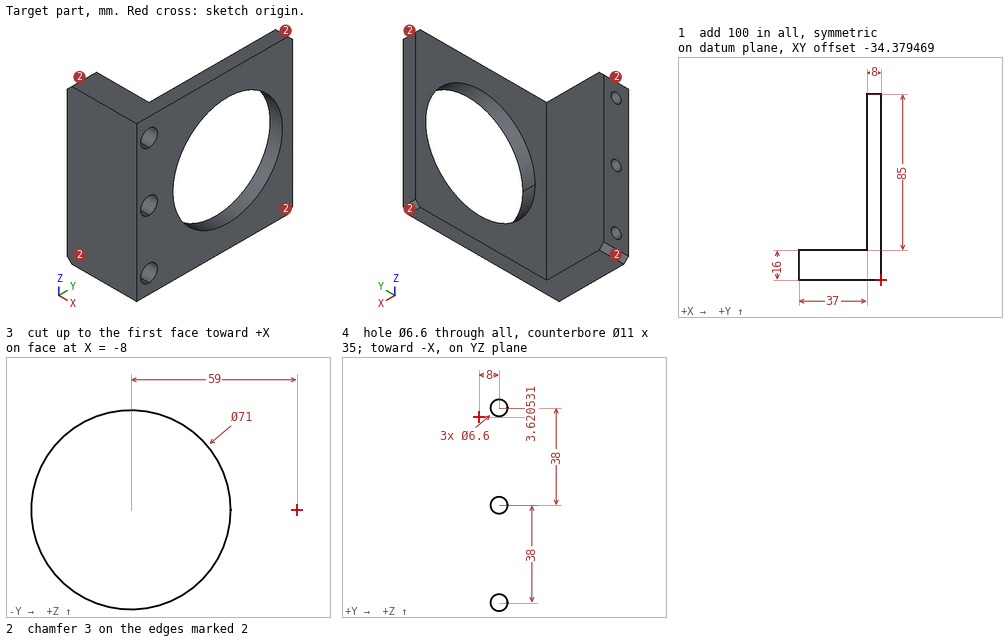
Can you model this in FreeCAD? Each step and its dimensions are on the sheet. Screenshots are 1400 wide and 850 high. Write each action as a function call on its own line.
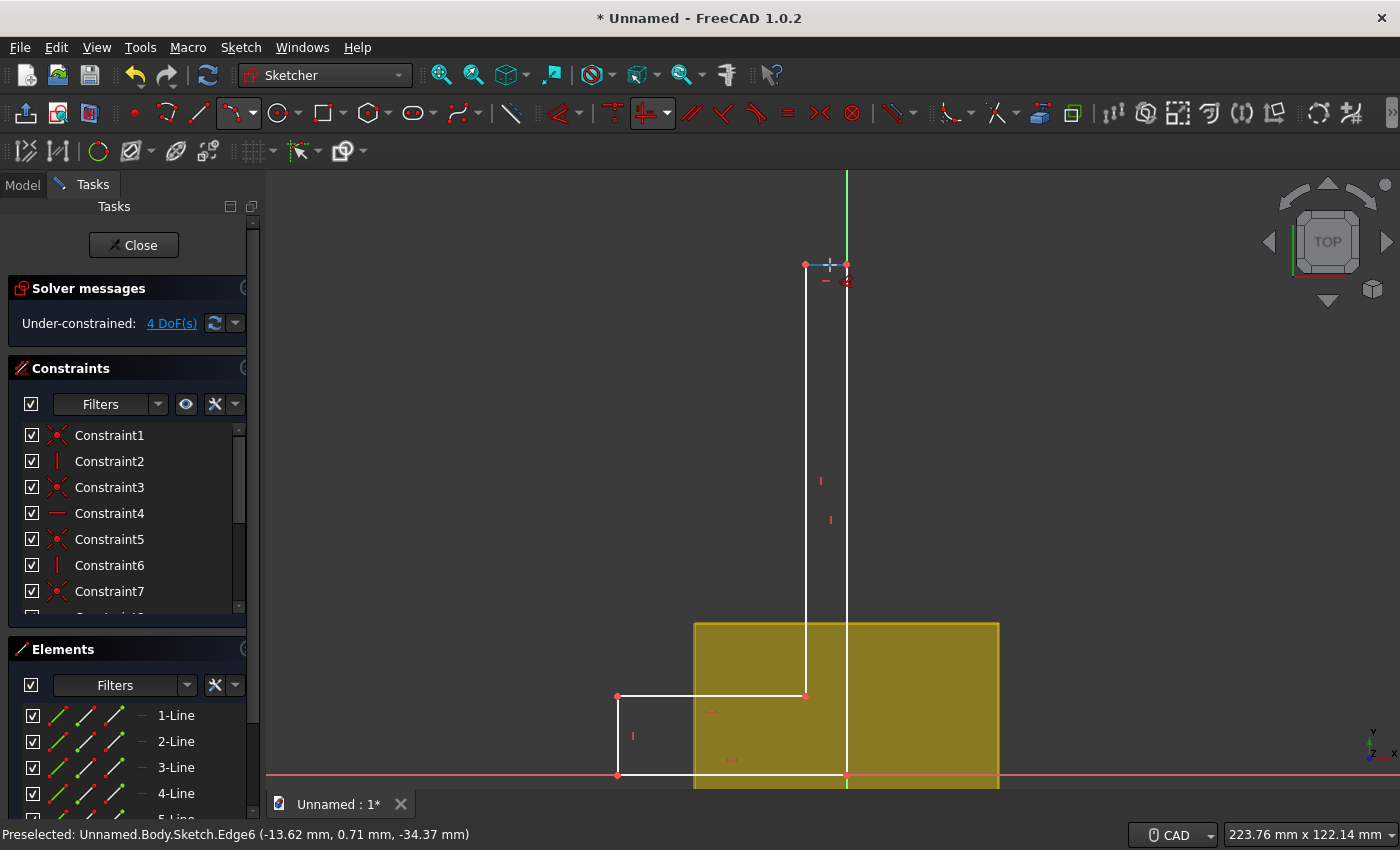
click(830, 265)
click(826, 231)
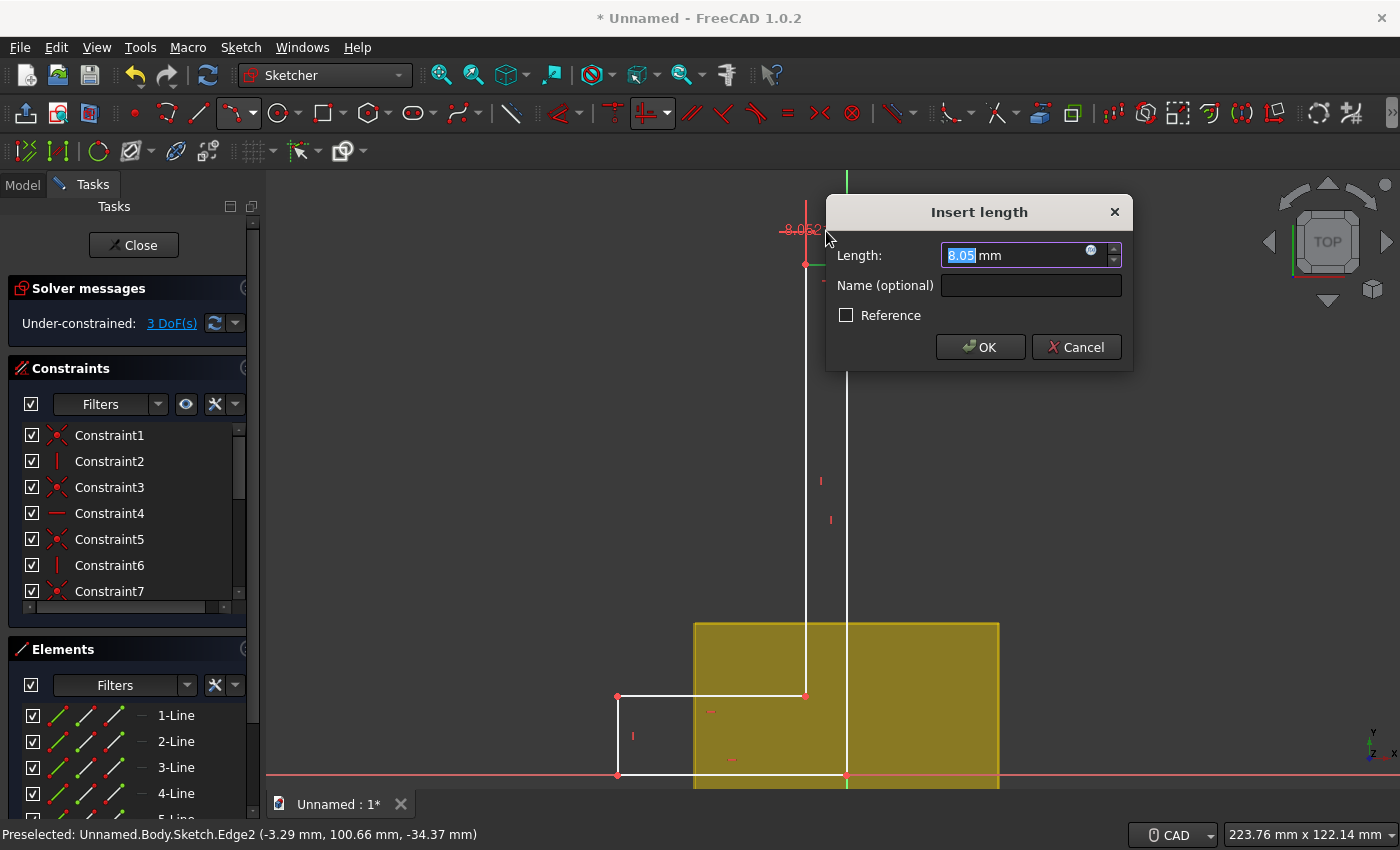
text(8)
key(Return)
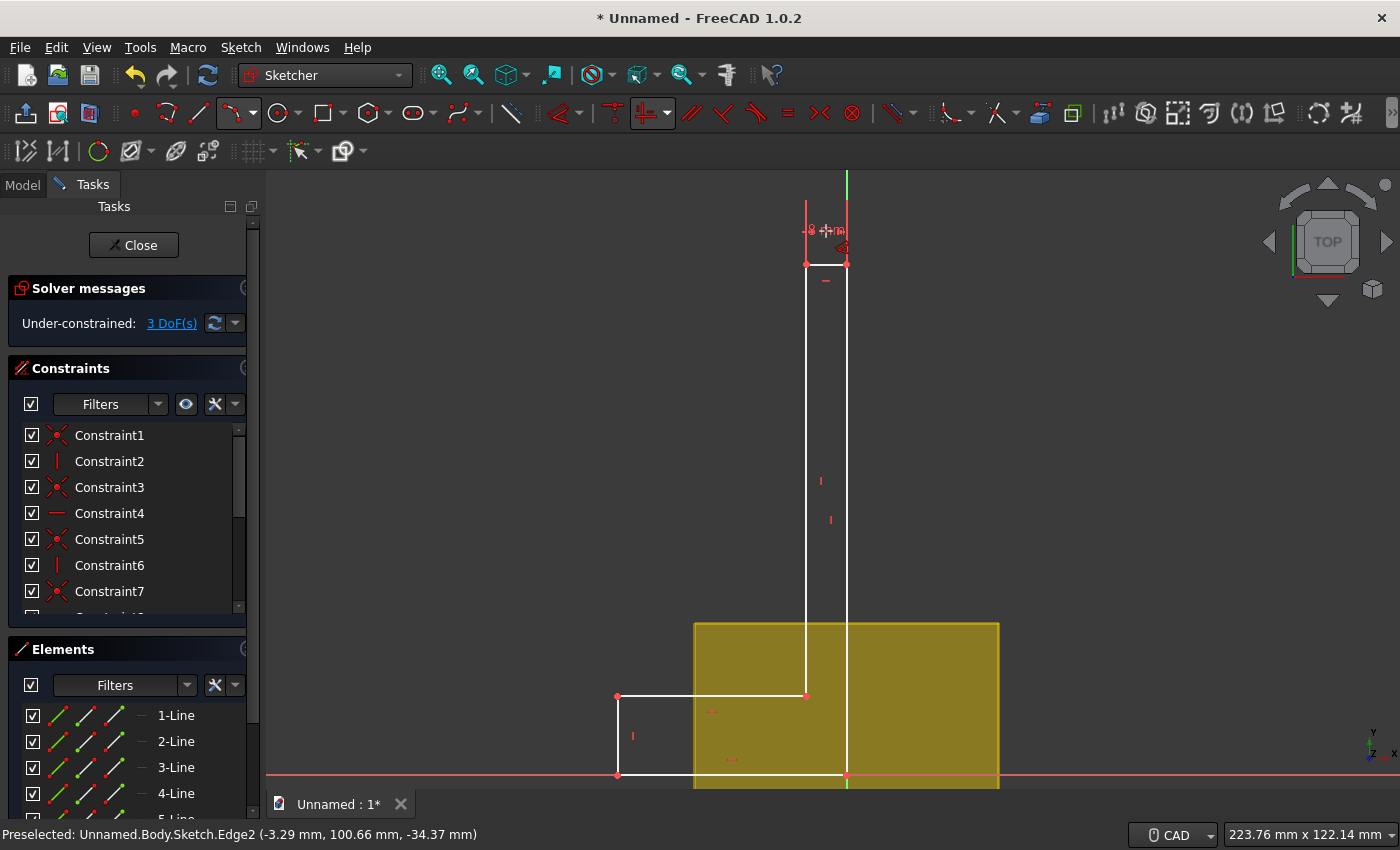
click(806, 394)
click(772, 480)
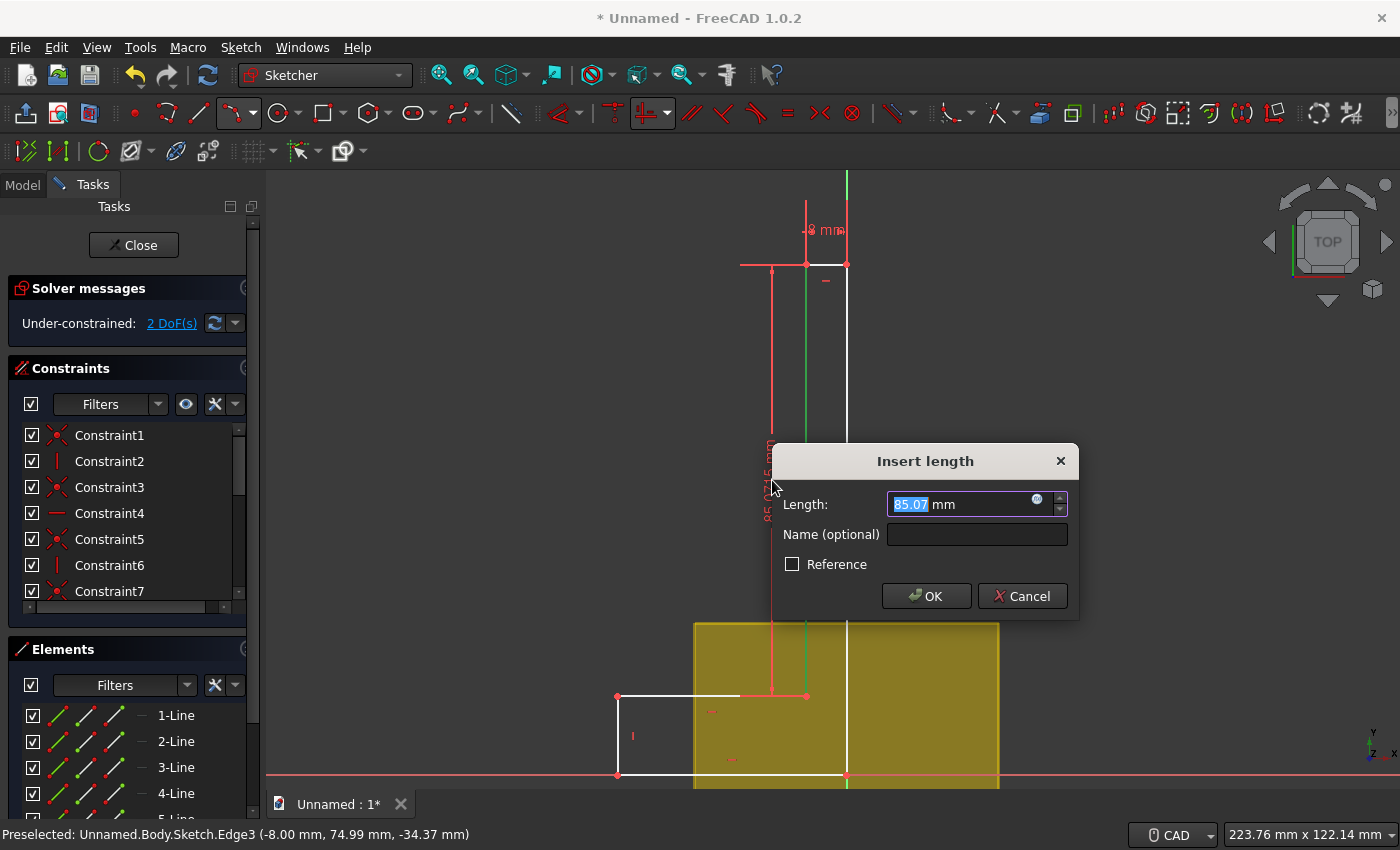
text(85)
key(Return)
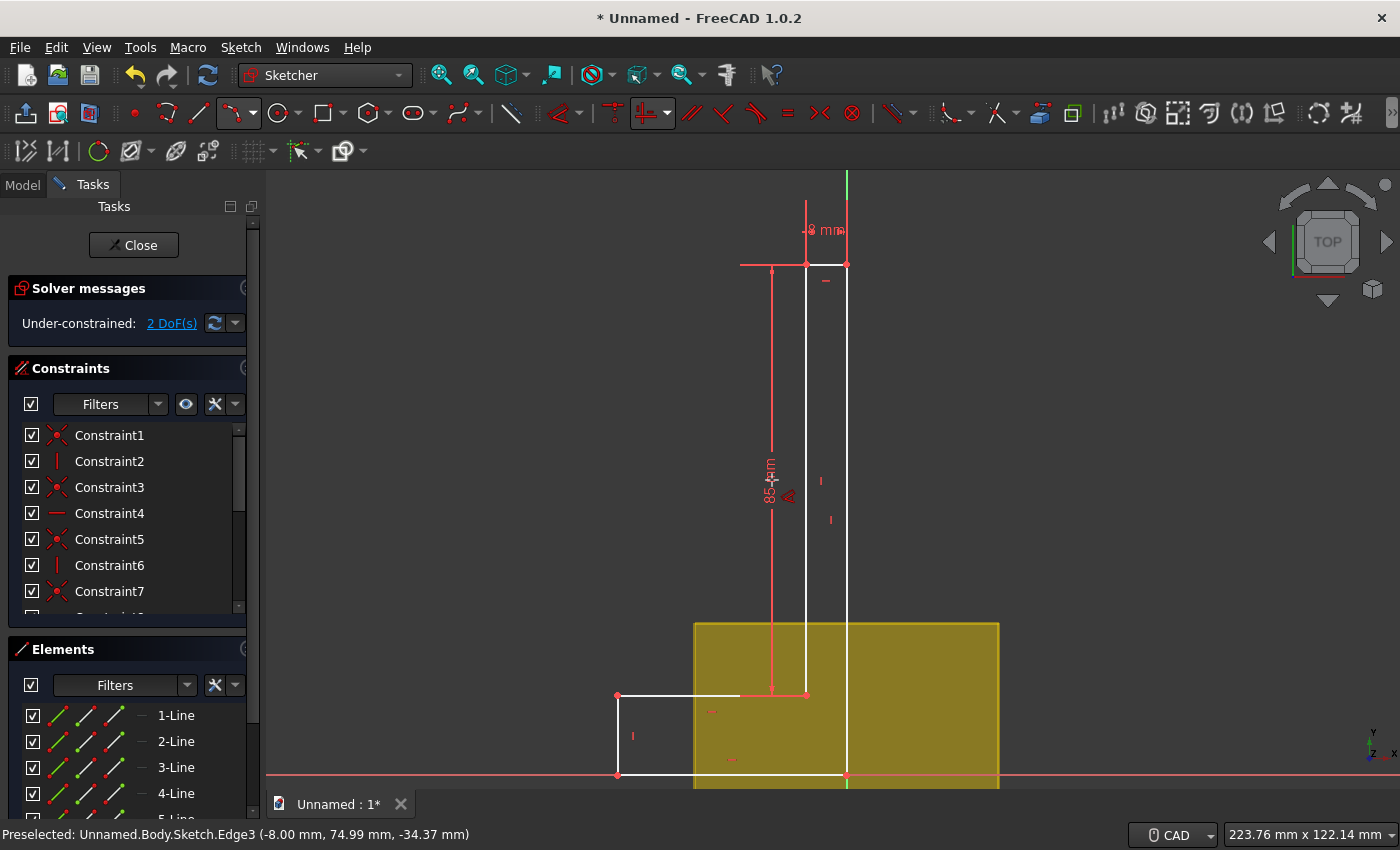
click(750, 696)
click(712, 730)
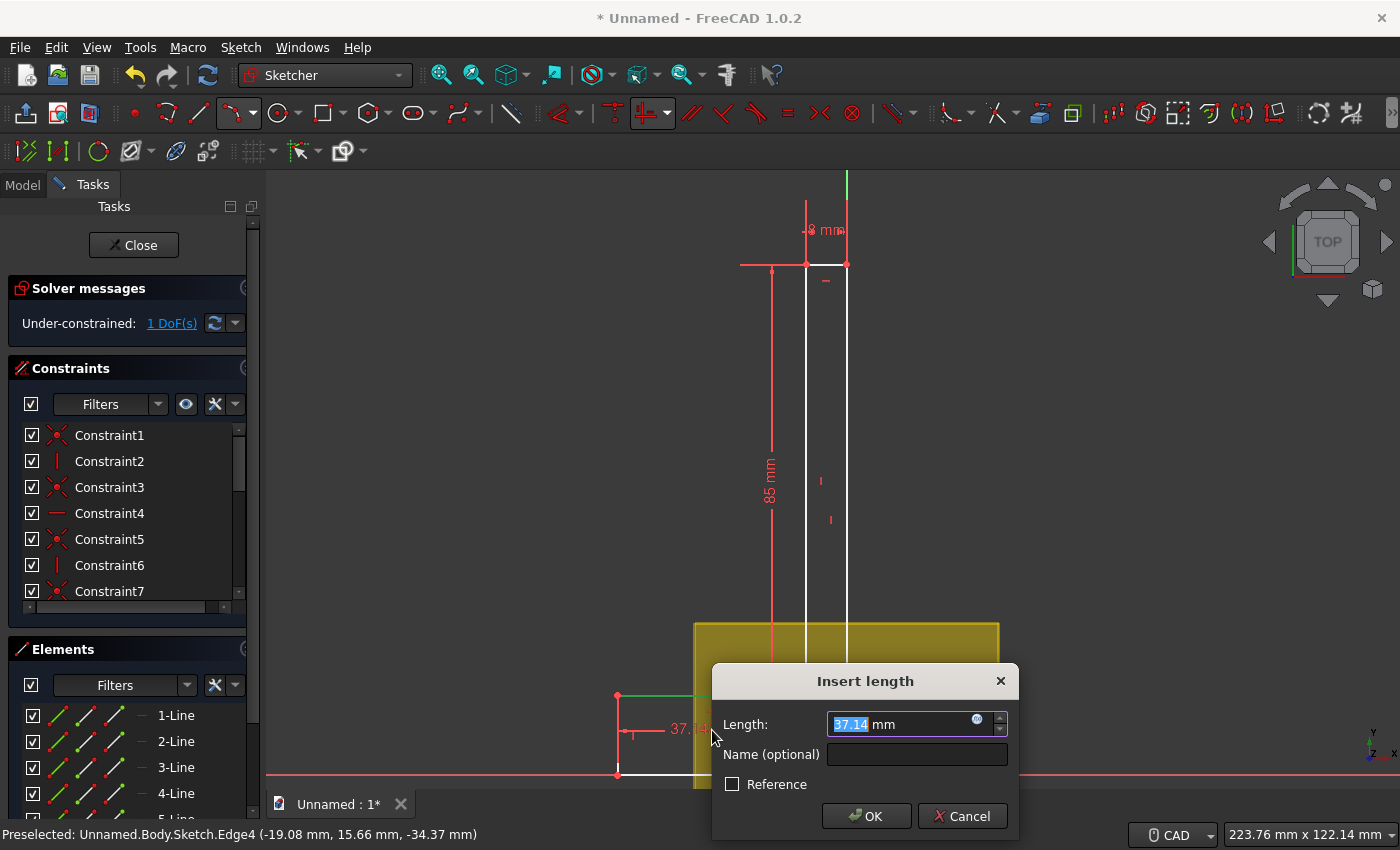
text(37)
key(Return)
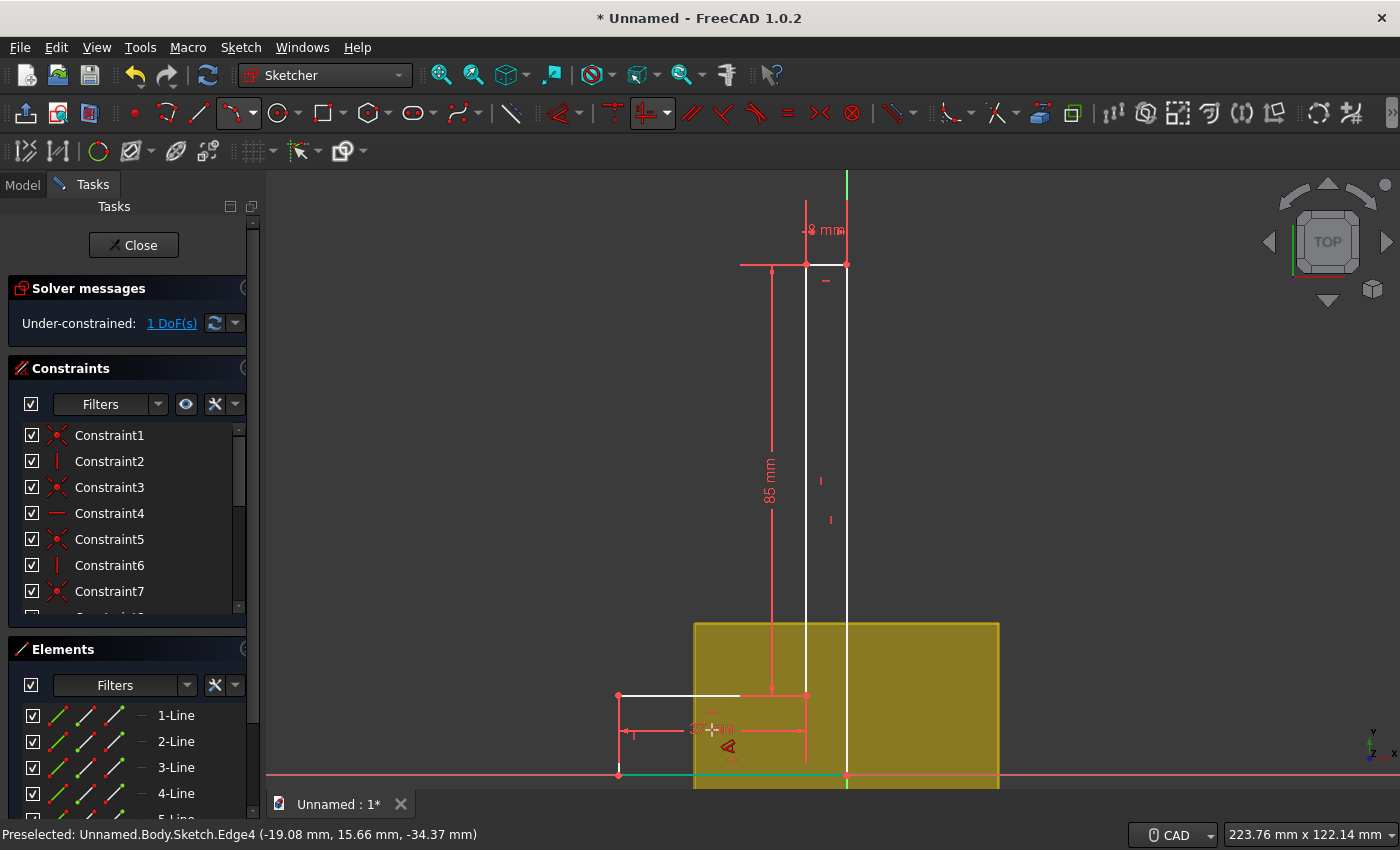
click(619, 720)
click(585, 728)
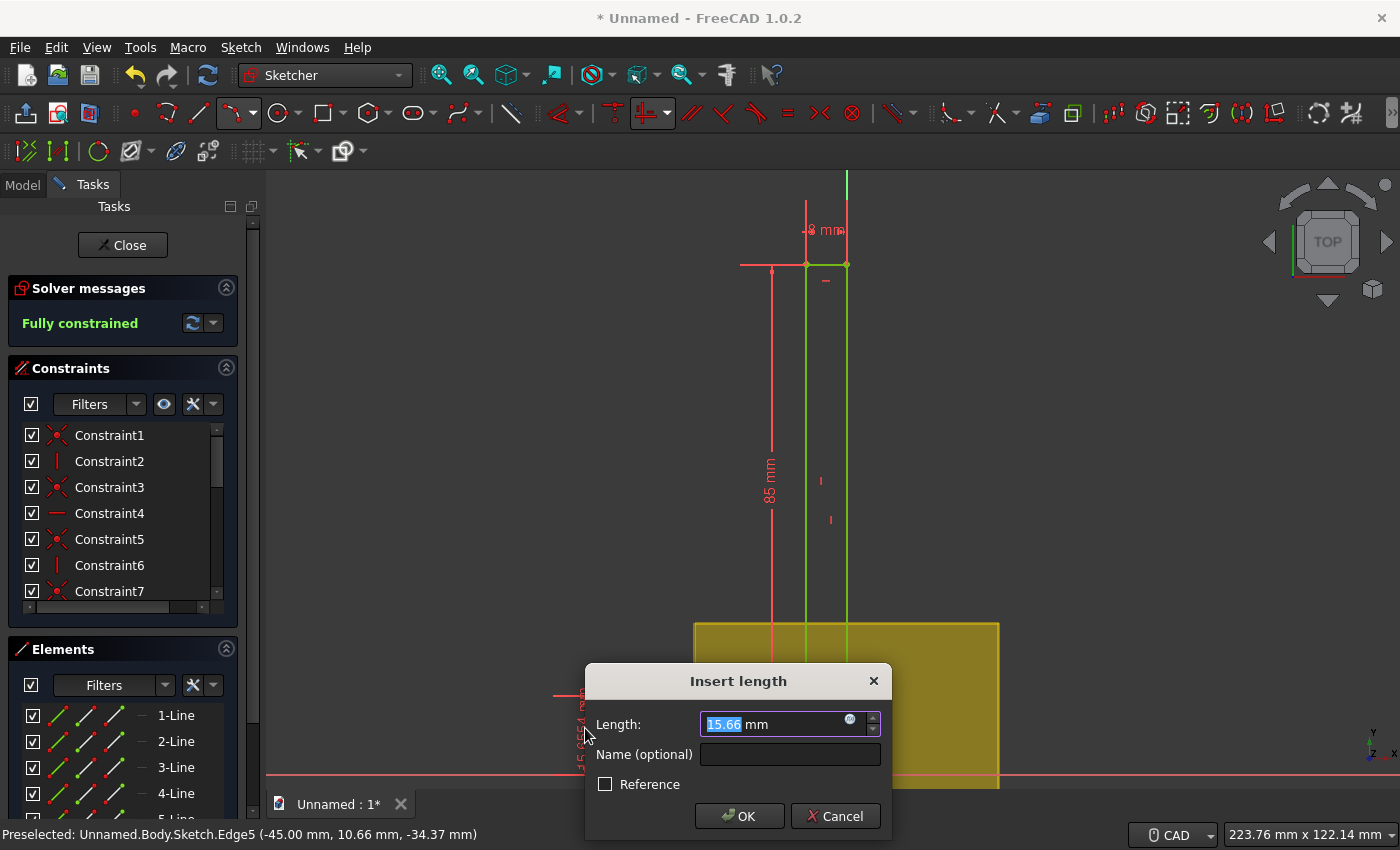
text(16)
key(Return)
key(Escape)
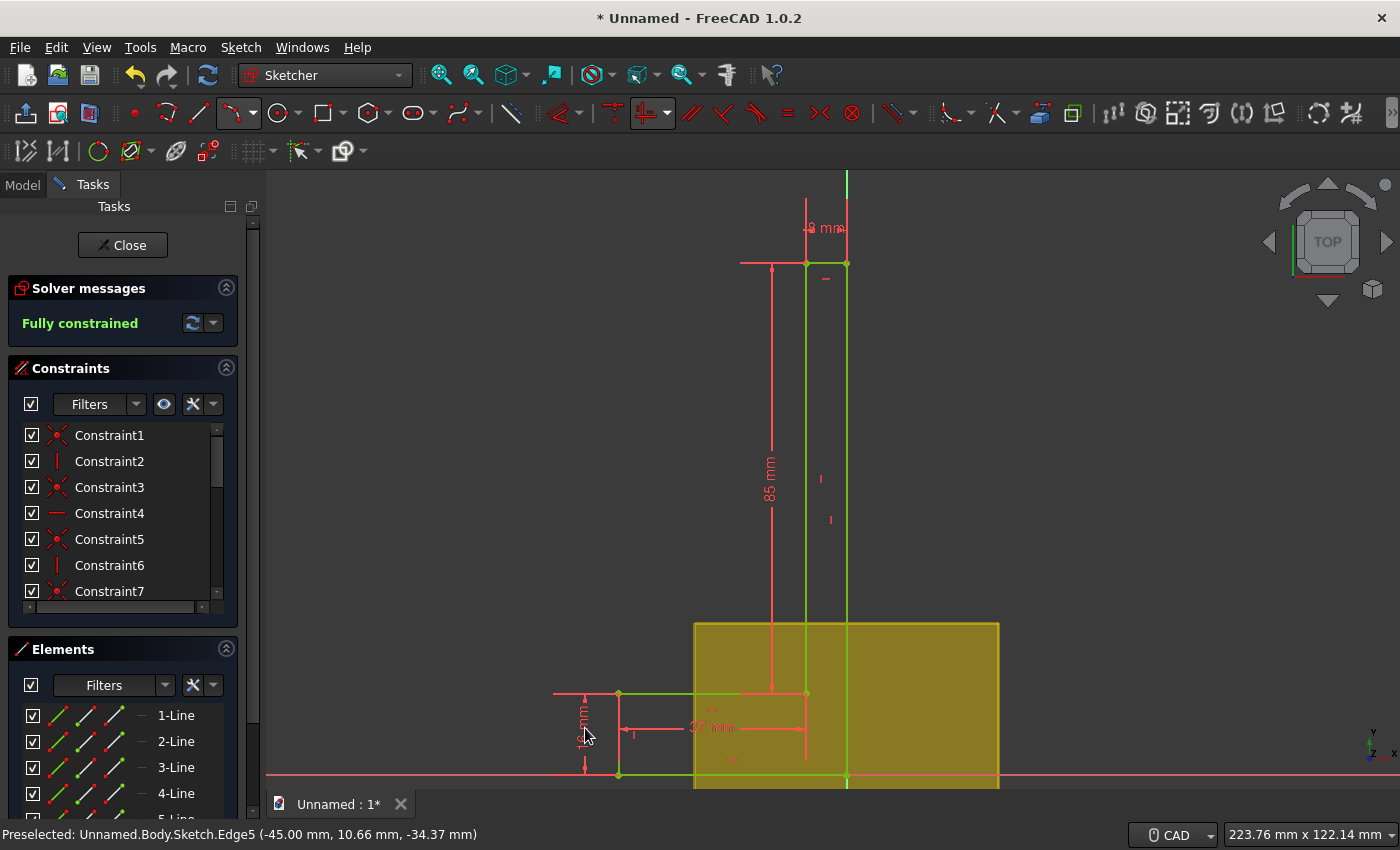
click(123, 245)